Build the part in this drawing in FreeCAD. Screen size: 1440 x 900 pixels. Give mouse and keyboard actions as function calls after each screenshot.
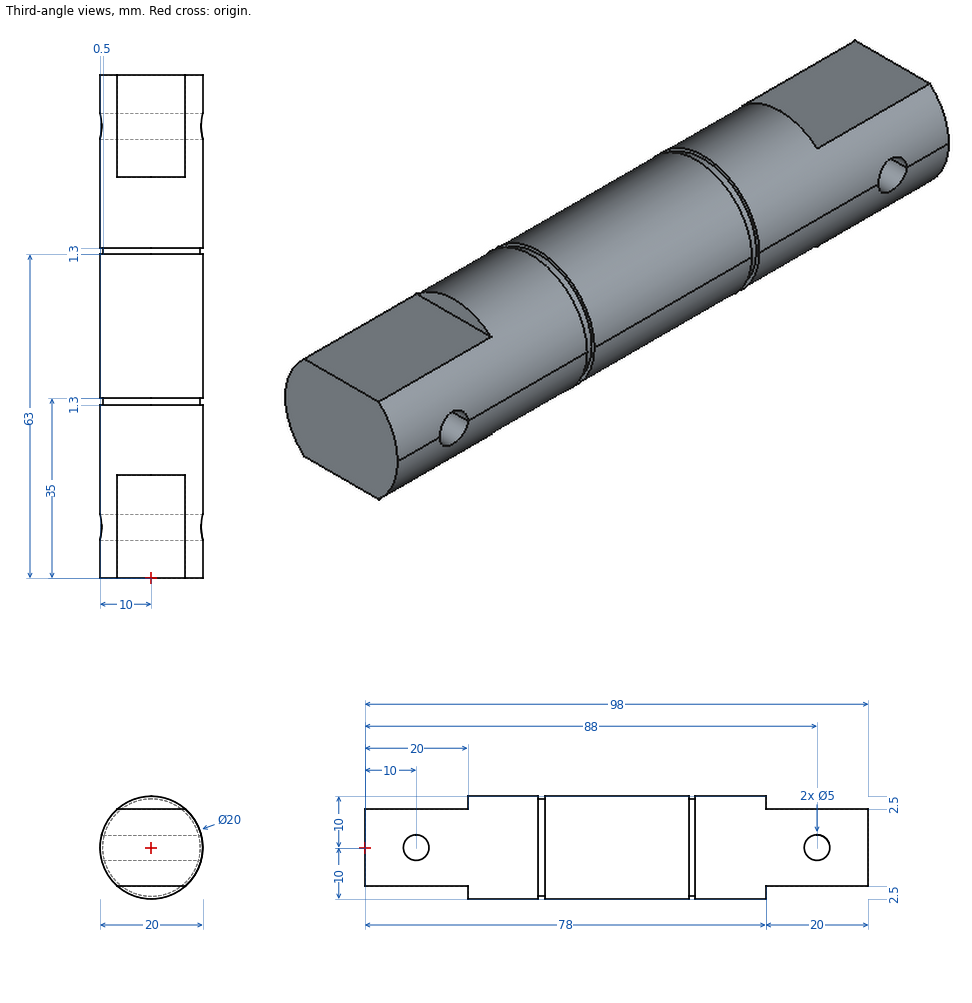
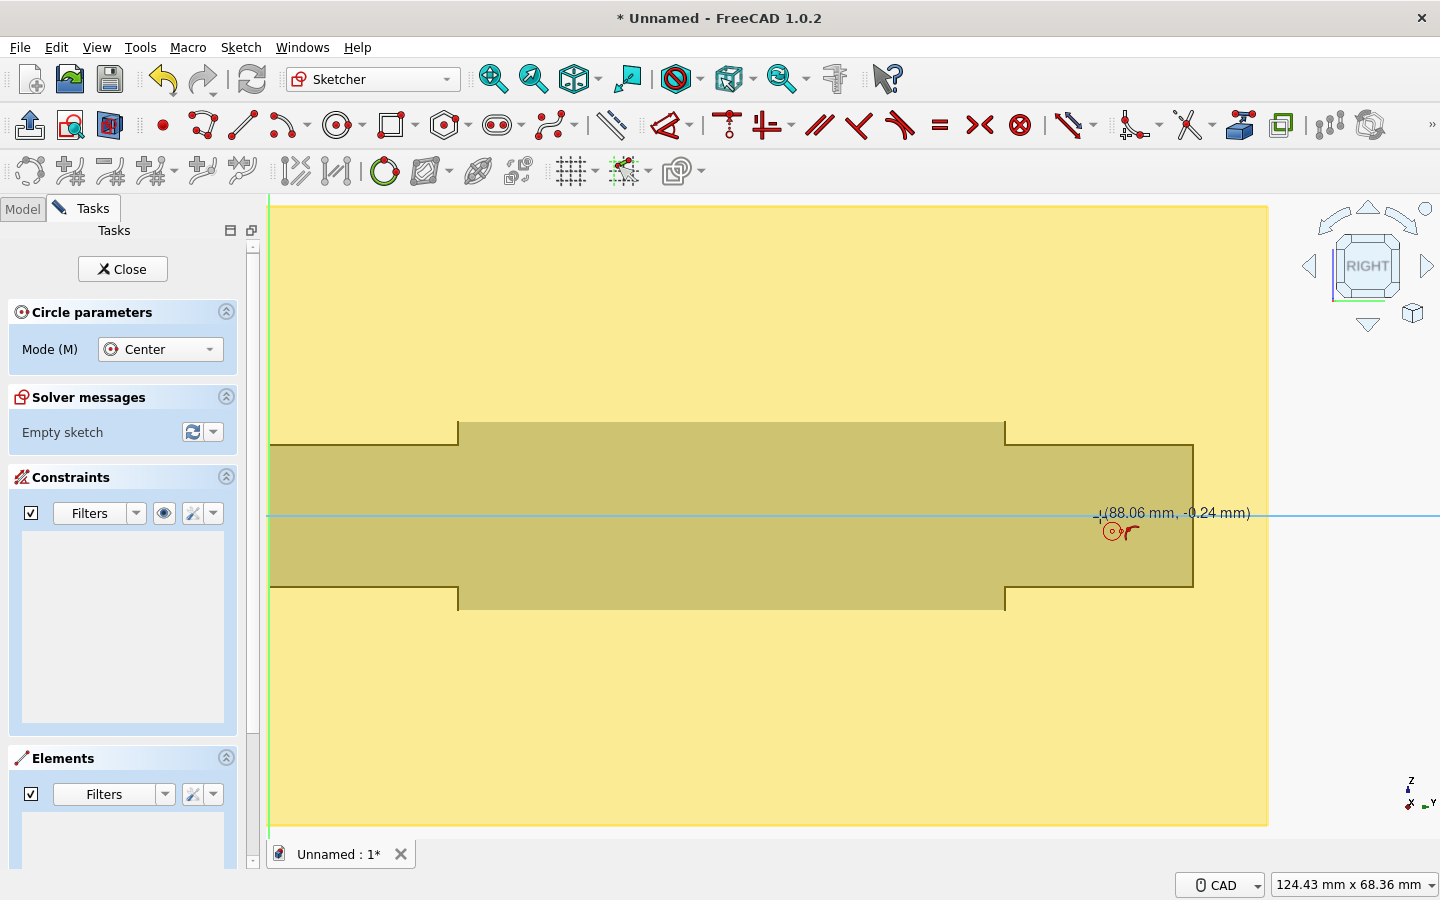
click(1099, 516)
move(1116, 499)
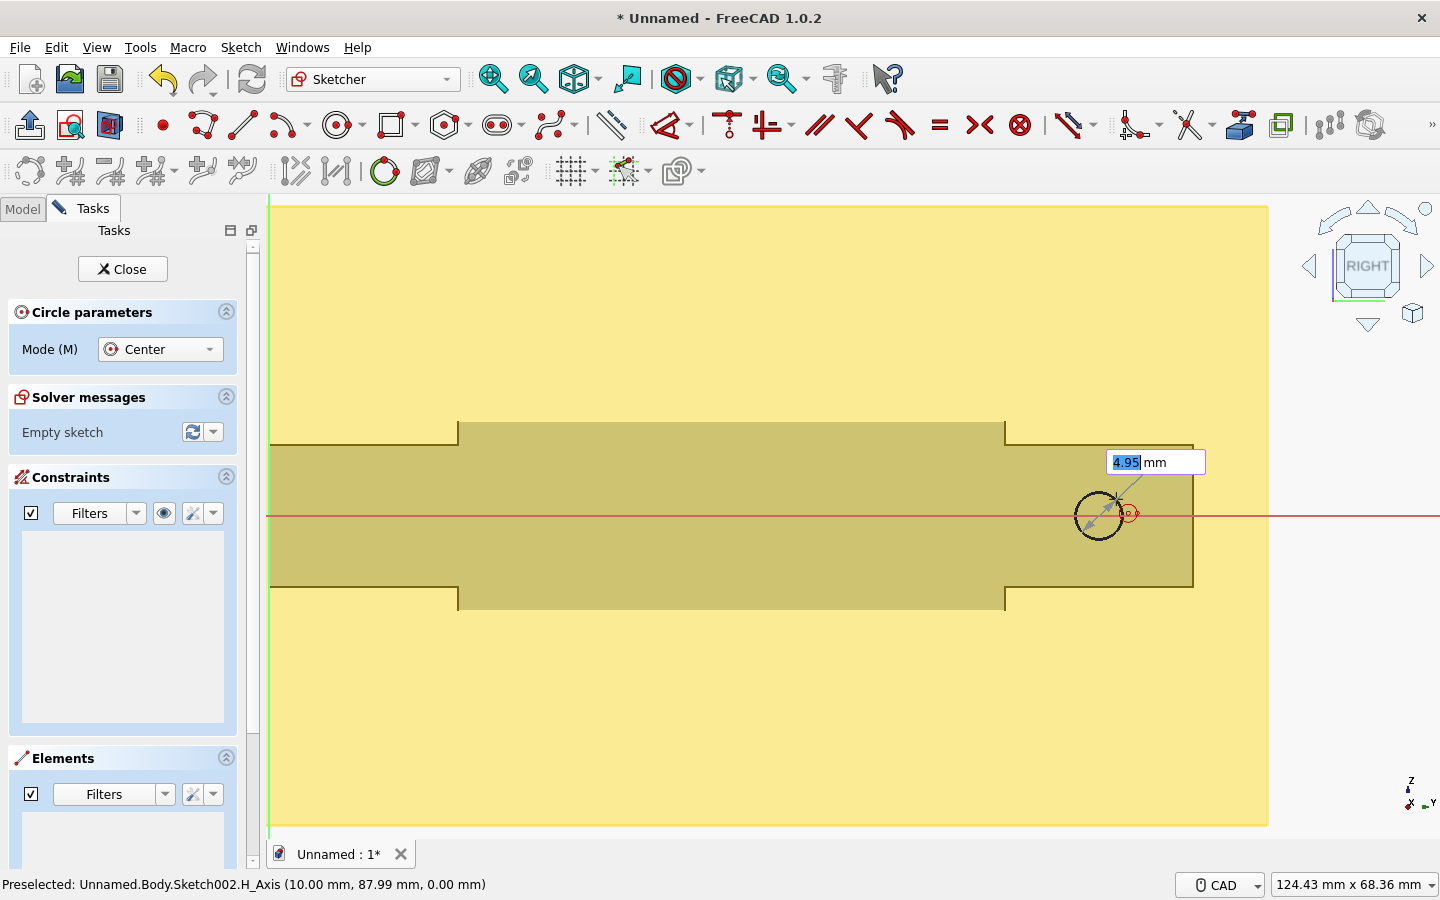
text(5)
key(Return)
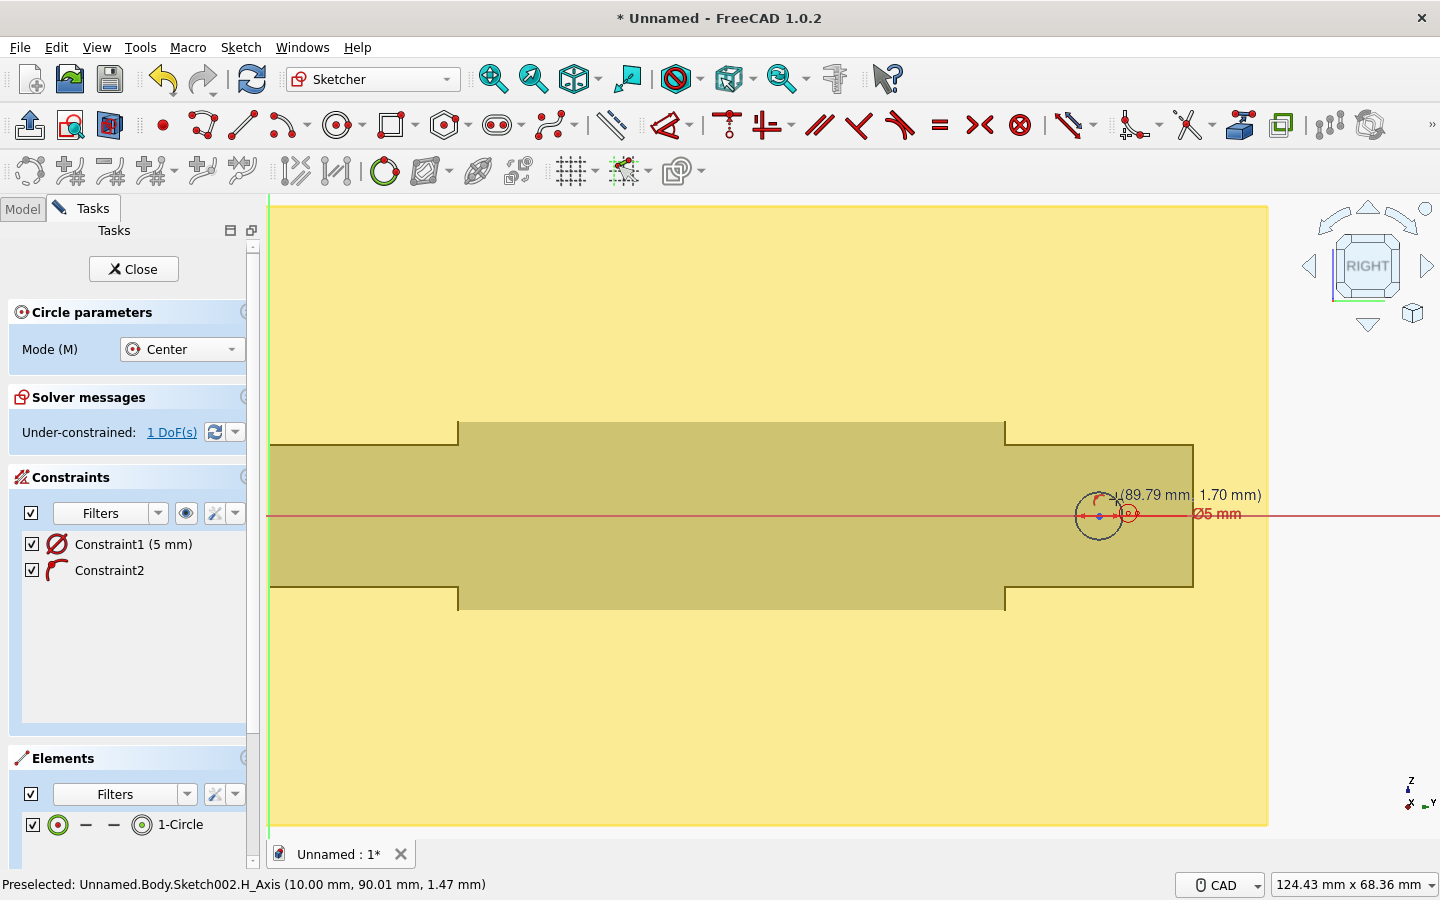
click(363, 516)
move(380, 499)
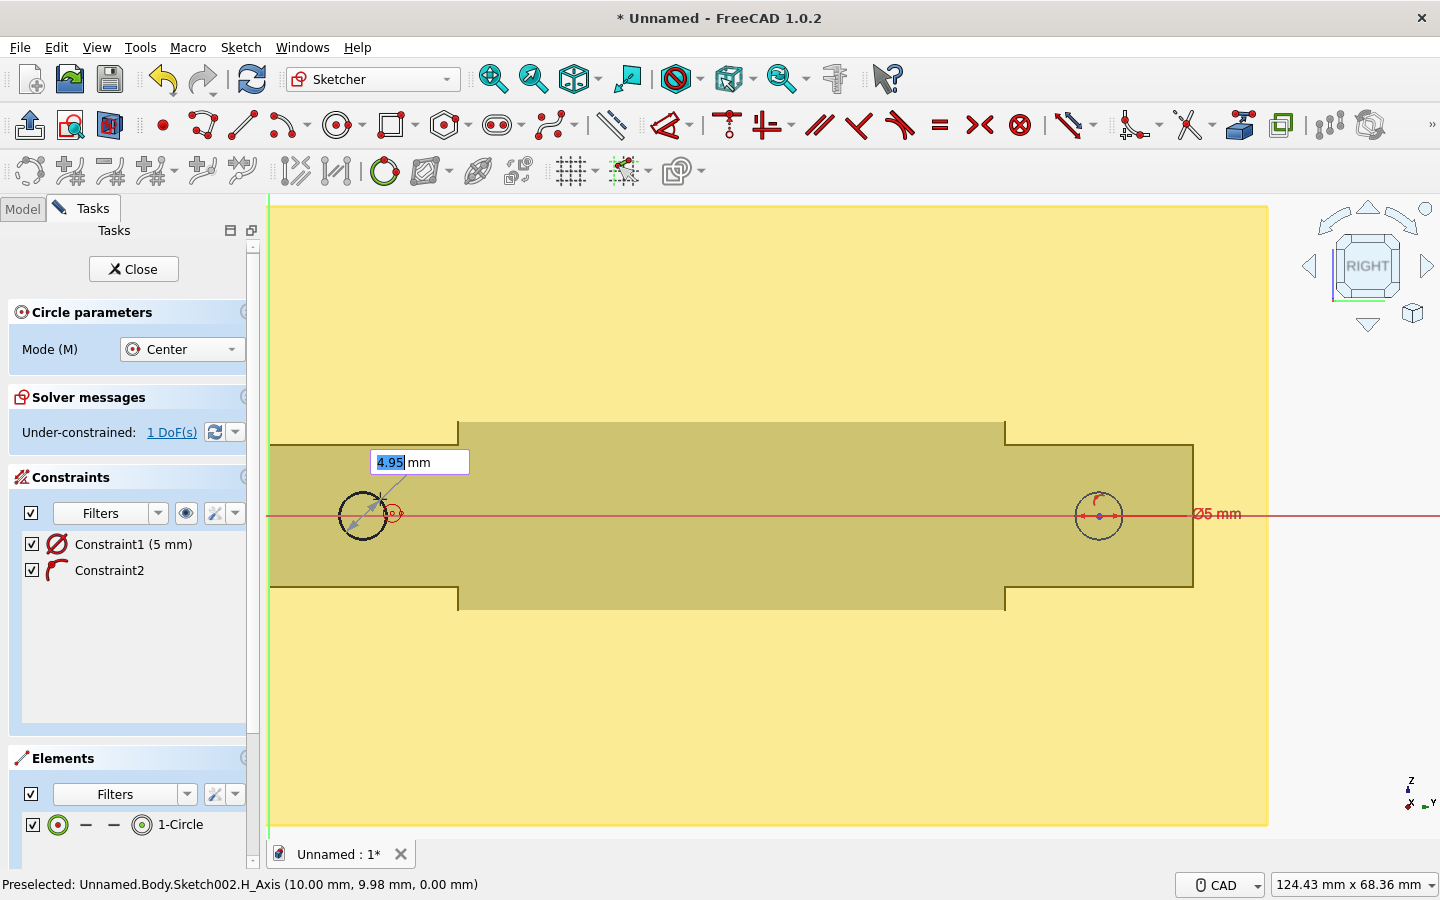
text(5)
key(Return)
key(Escape)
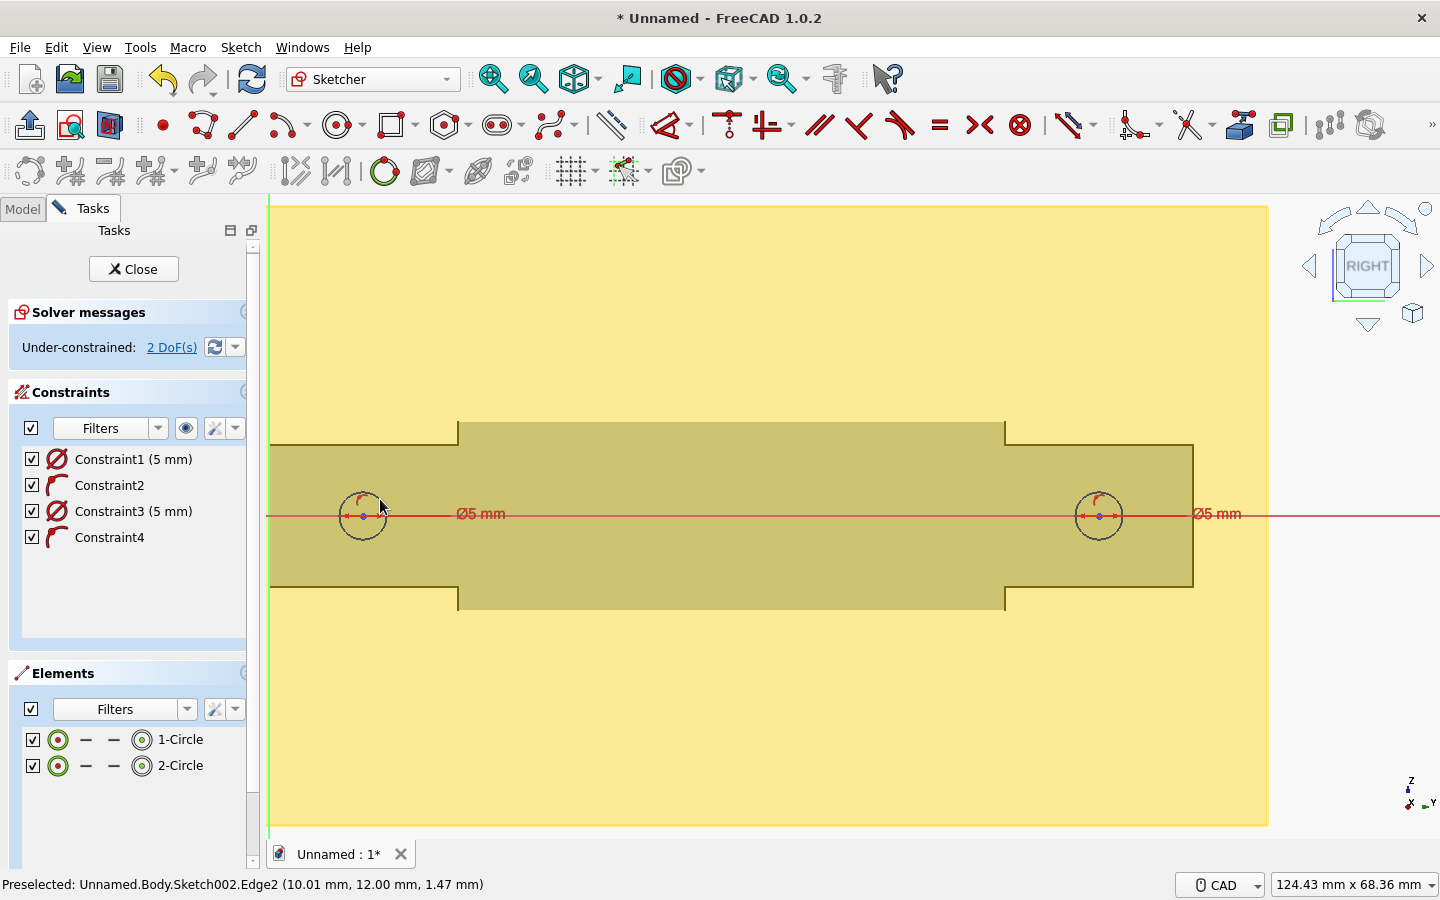
key(d)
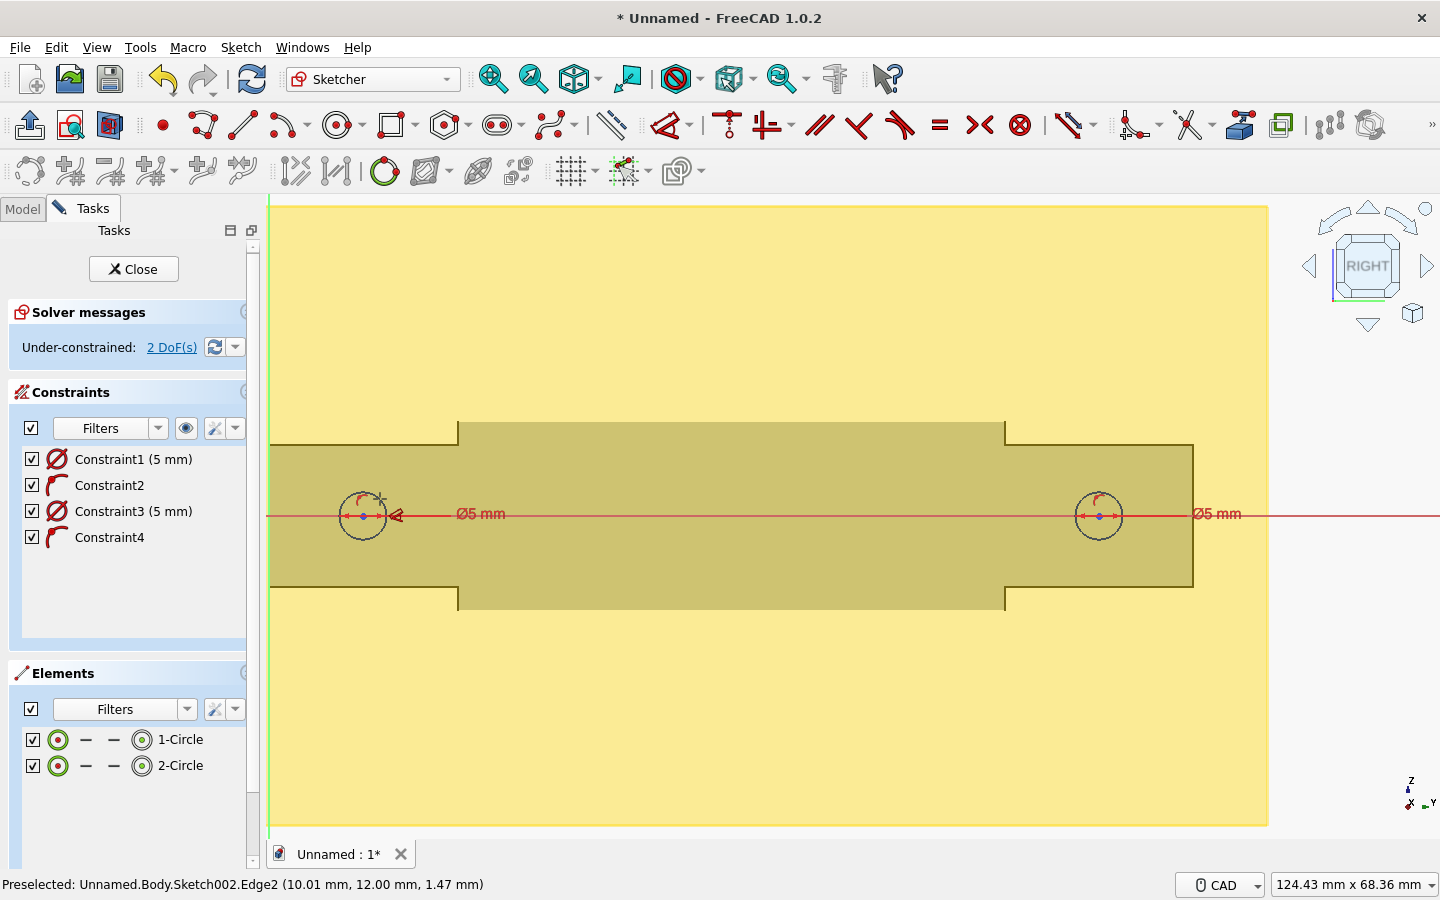
click(1099, 516)
click(696, 550)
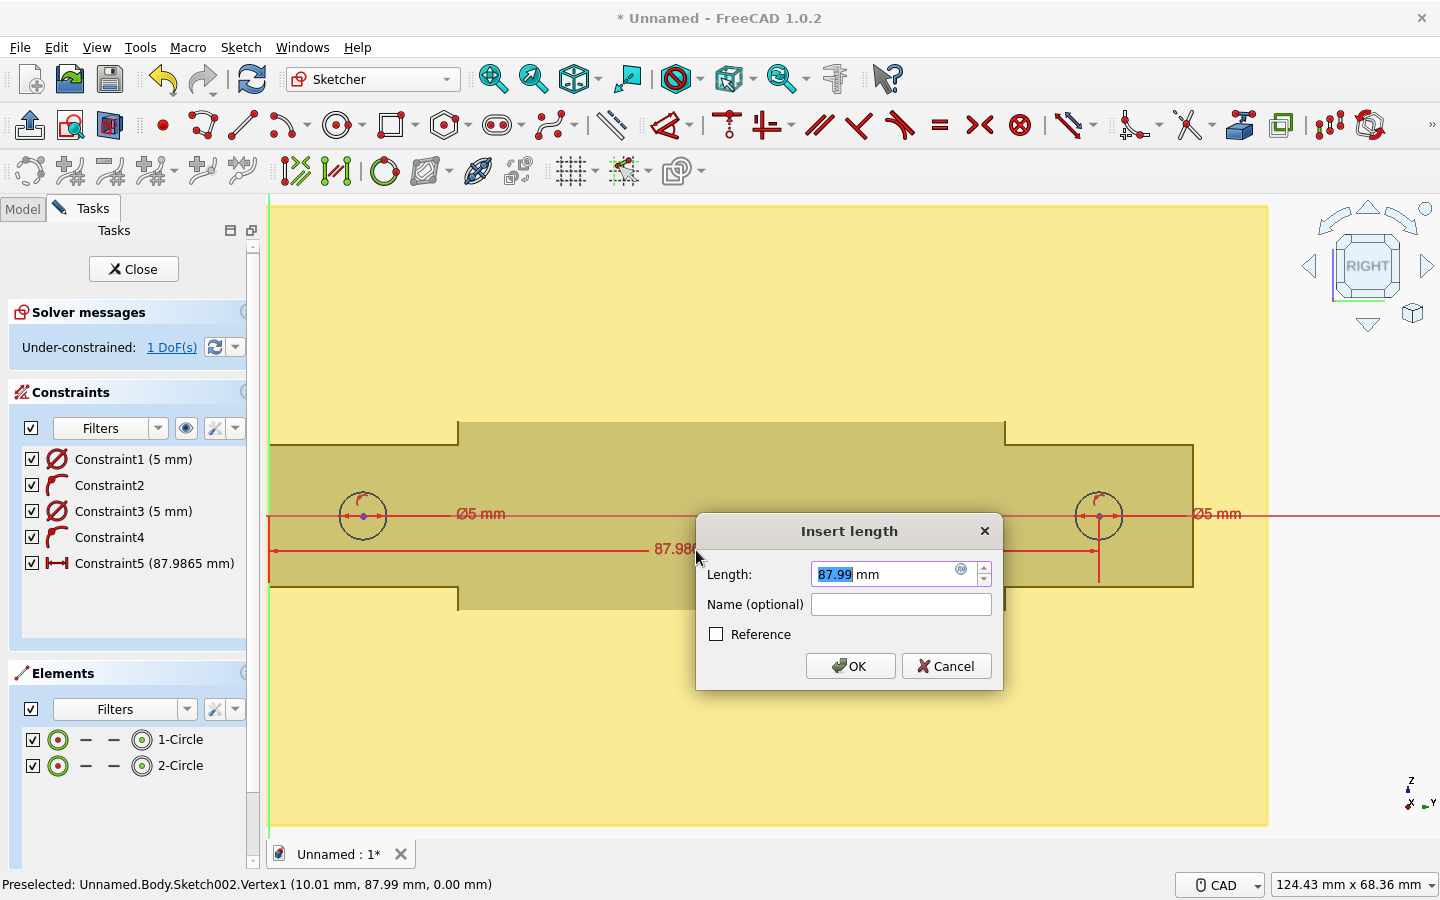
text(88)
key(Return)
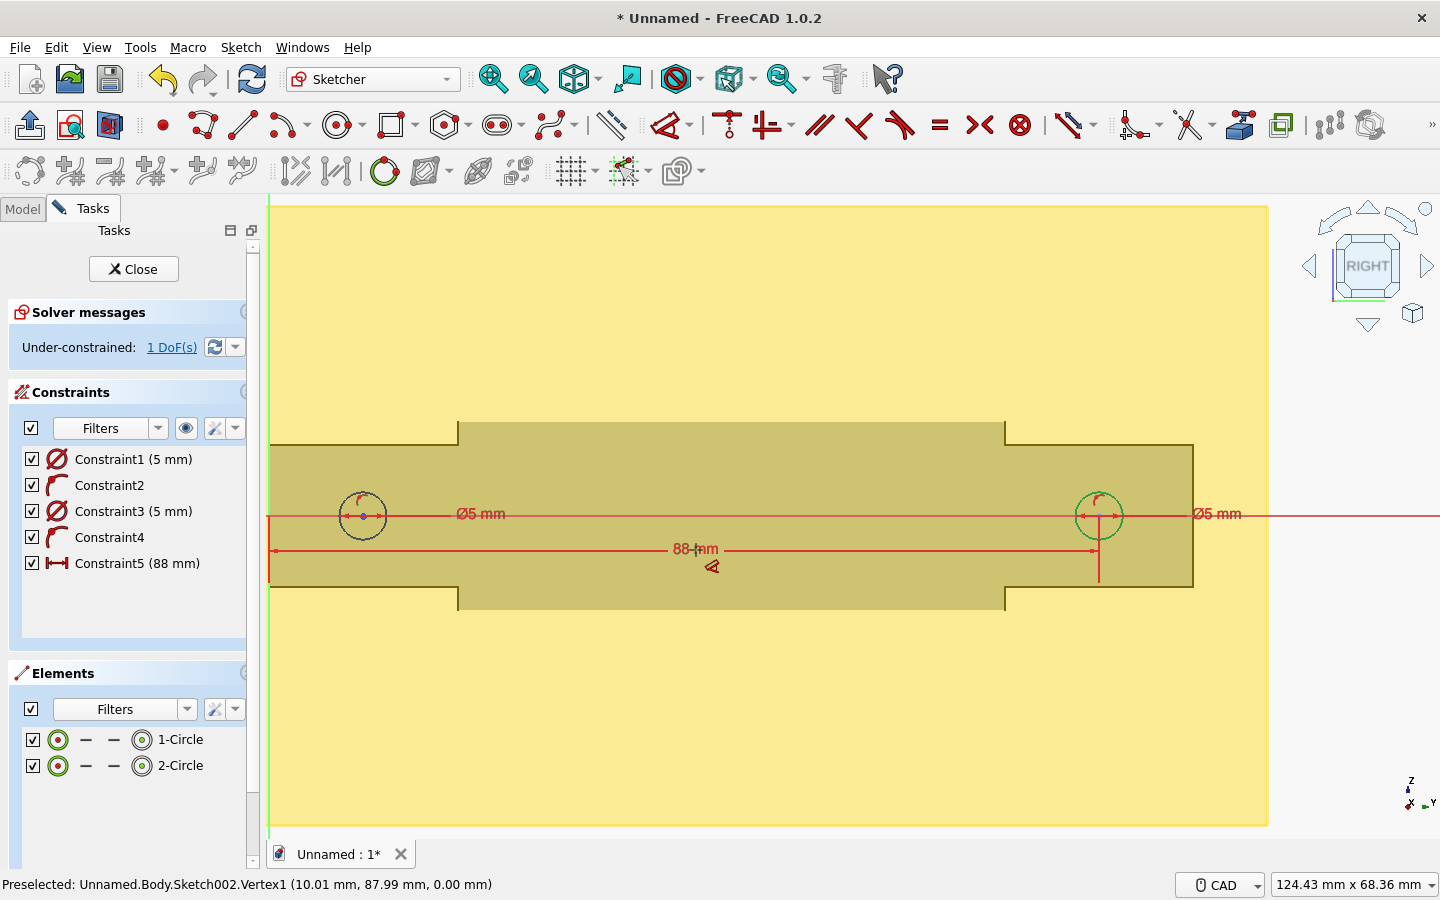
click(363, 516)
click(329, 550)